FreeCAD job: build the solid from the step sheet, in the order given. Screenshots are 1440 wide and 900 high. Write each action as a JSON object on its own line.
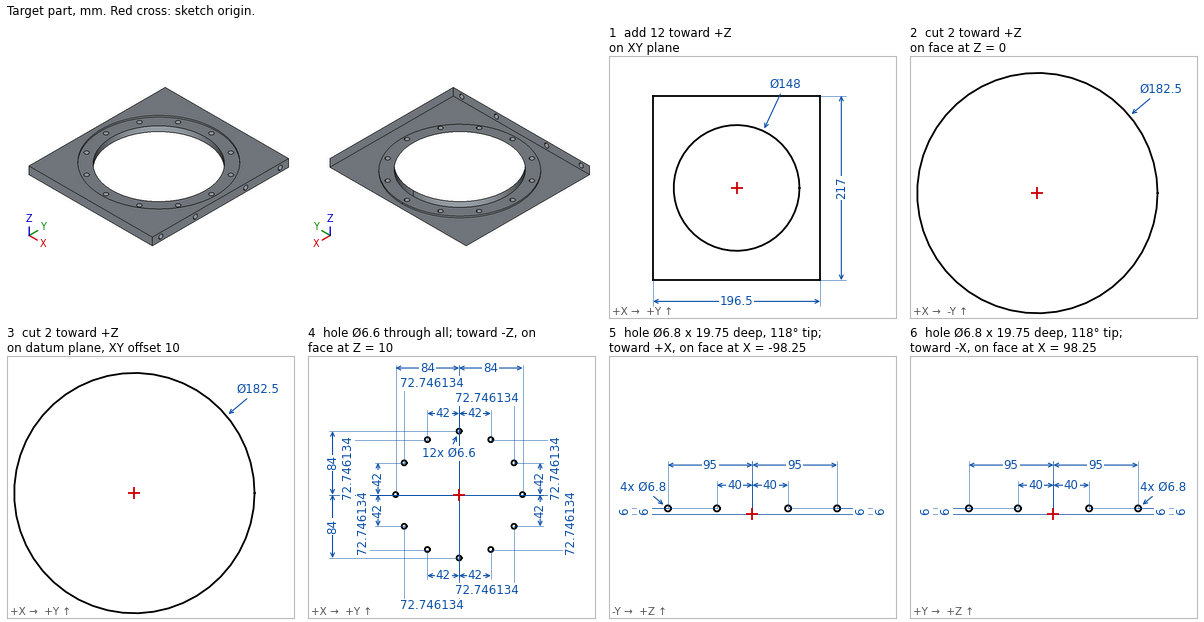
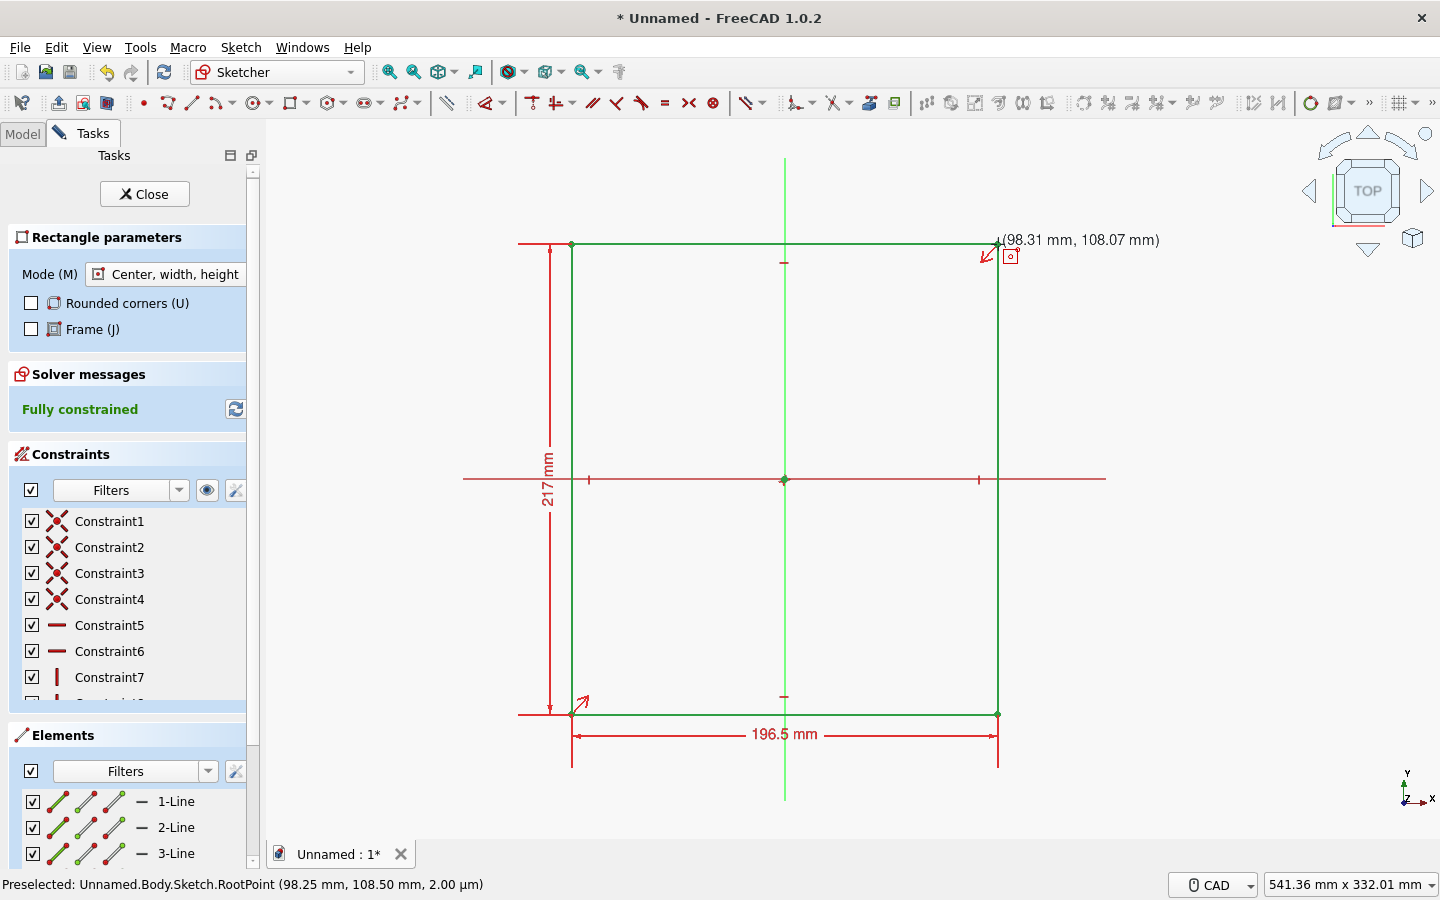
{"action": "left_click", "coordinate": [254, 104]}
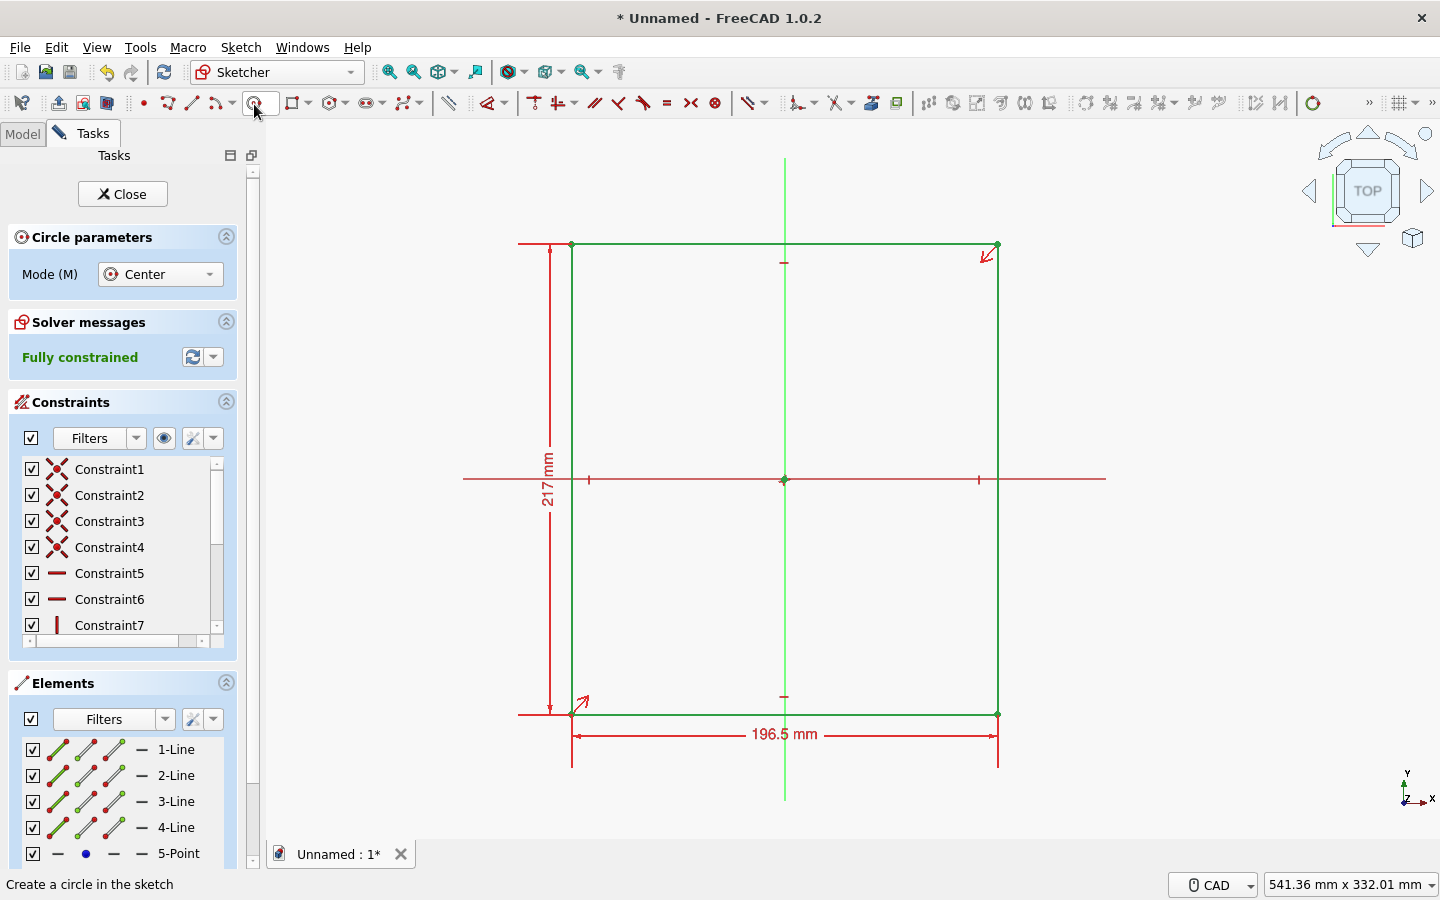
{"action": "left_click", "coordinate": [785, 479]}
{"action": "mouse_move", "coordinate": [898, 366]}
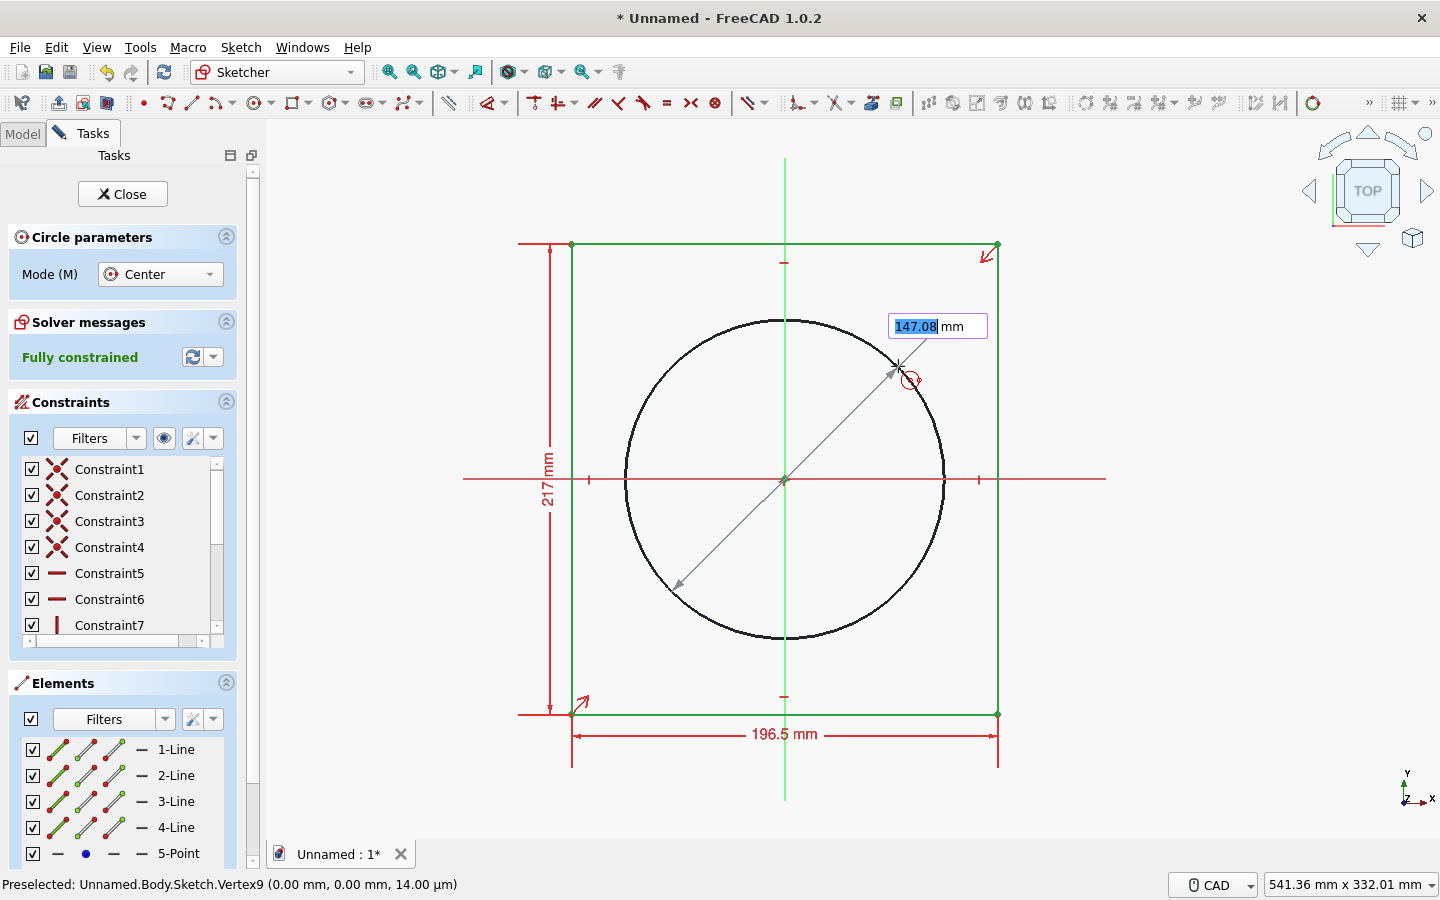
{"action": "type", "text": "148"}
{"action": "key", "text": "Return"}
{"action": "key", "text": "Escape"}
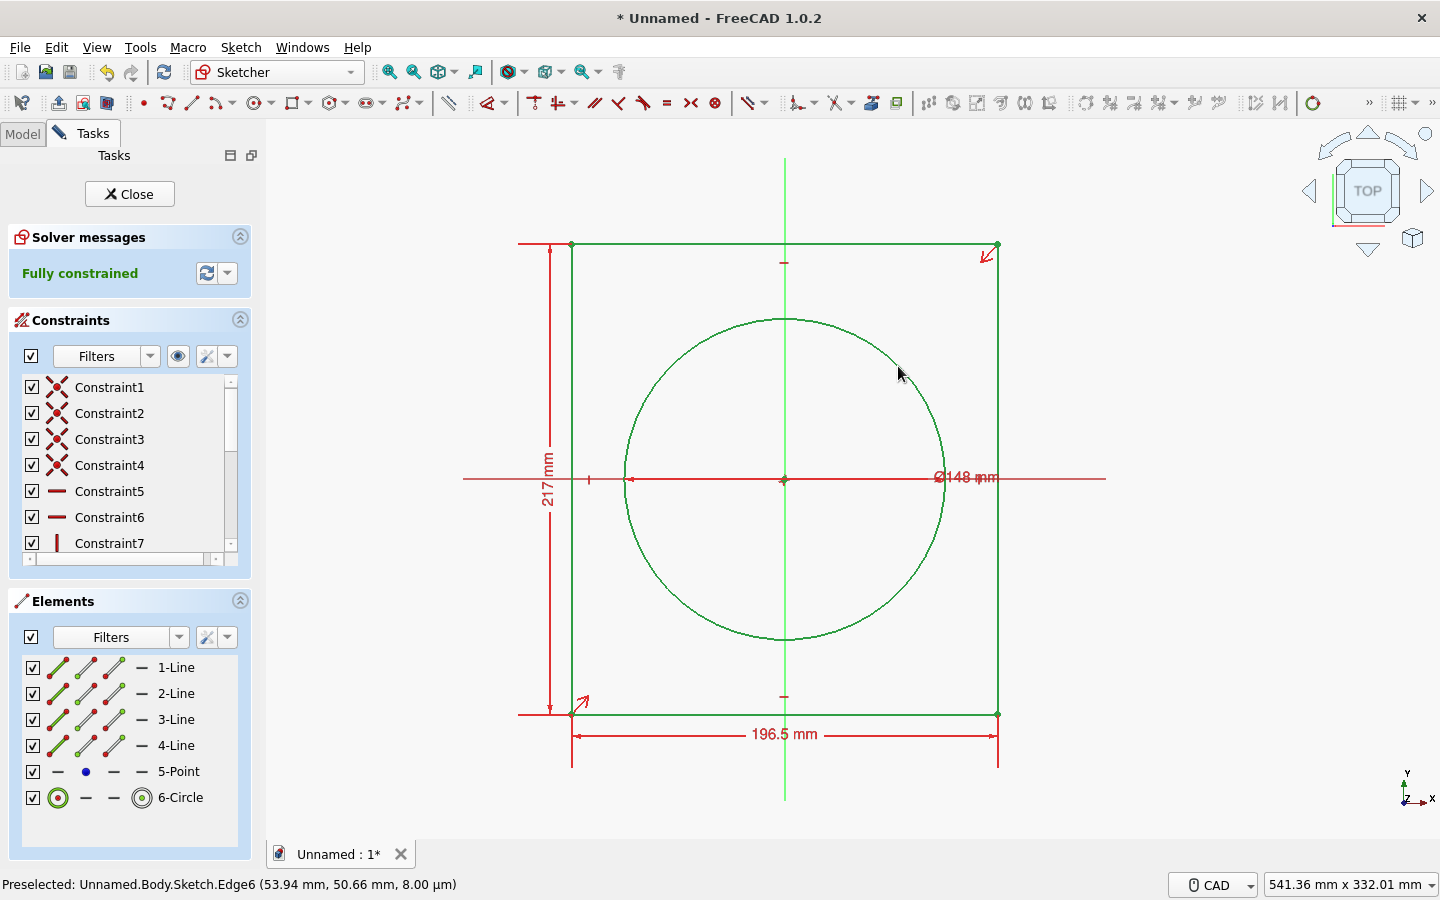
{"action": "left_click", "coordinate": [130, 194]}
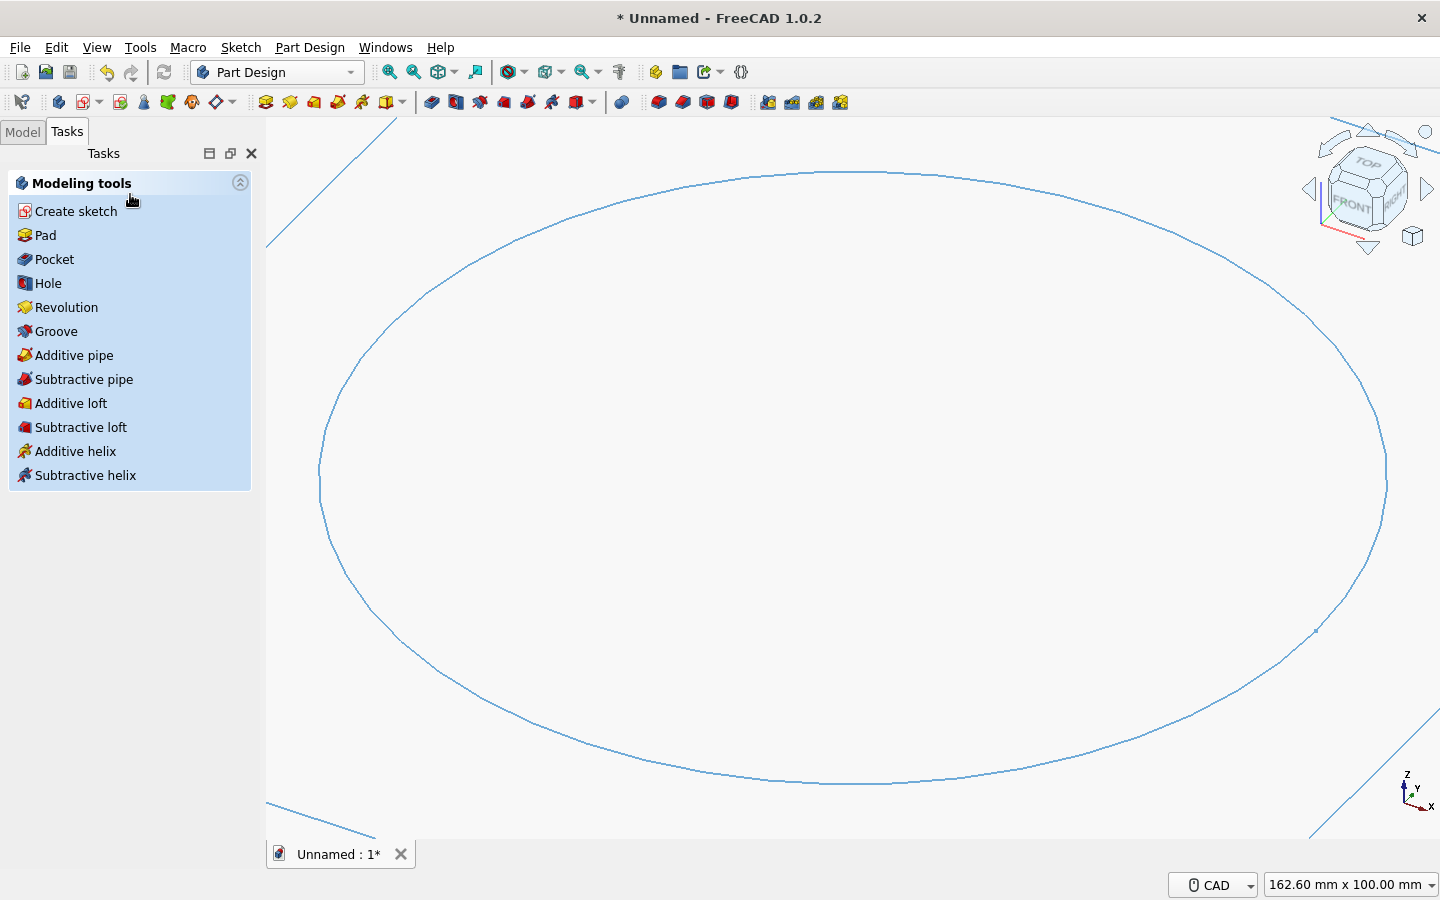
{"action": "left_click", "coordinate": [266, 102]}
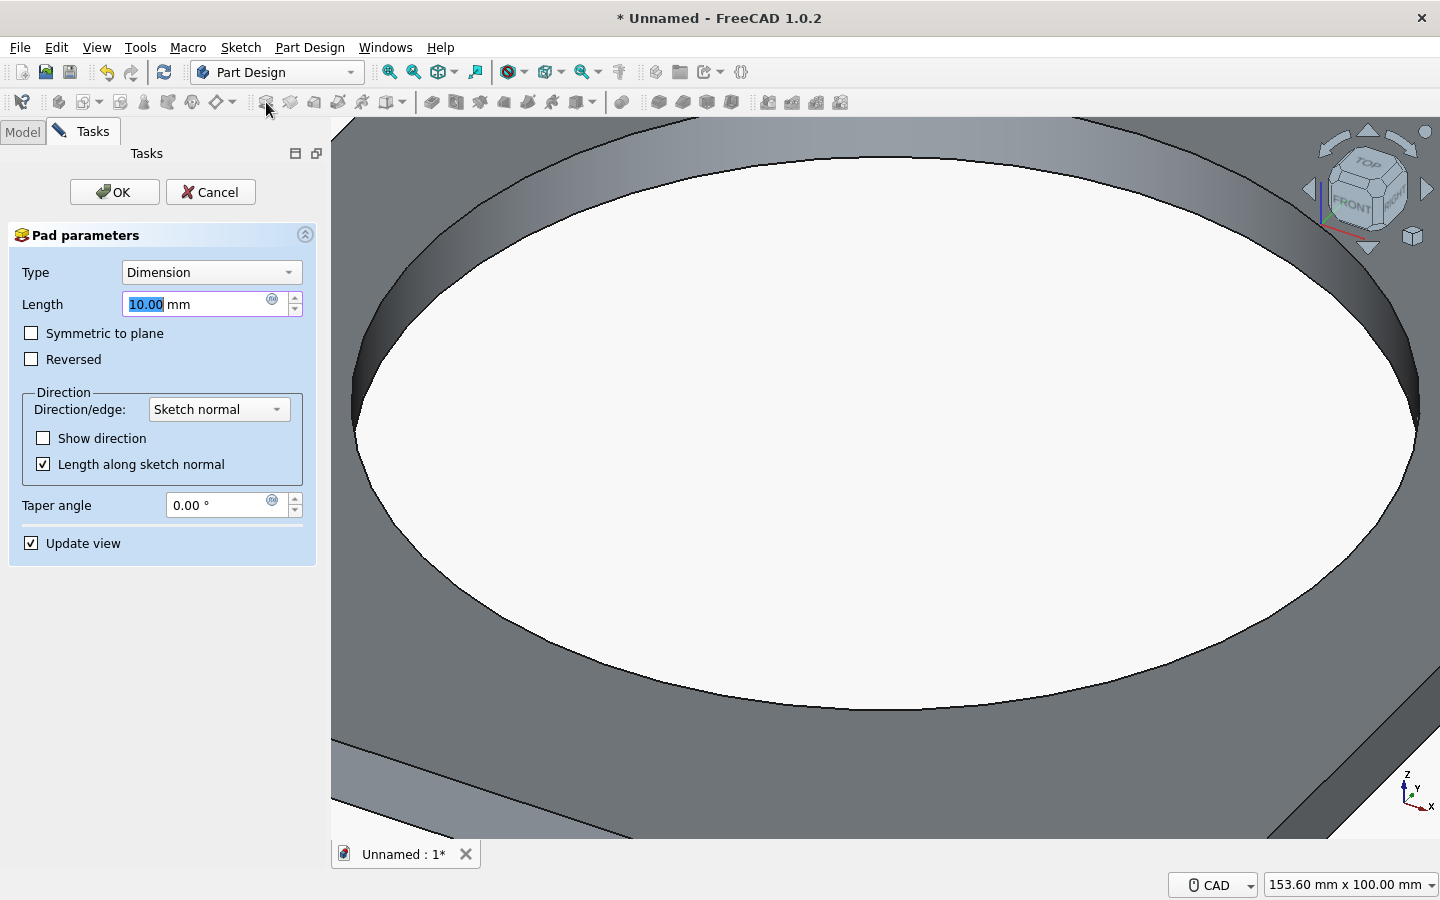
{"action": "type", "text": "12"}
{"action": "key", "text": "Tab"}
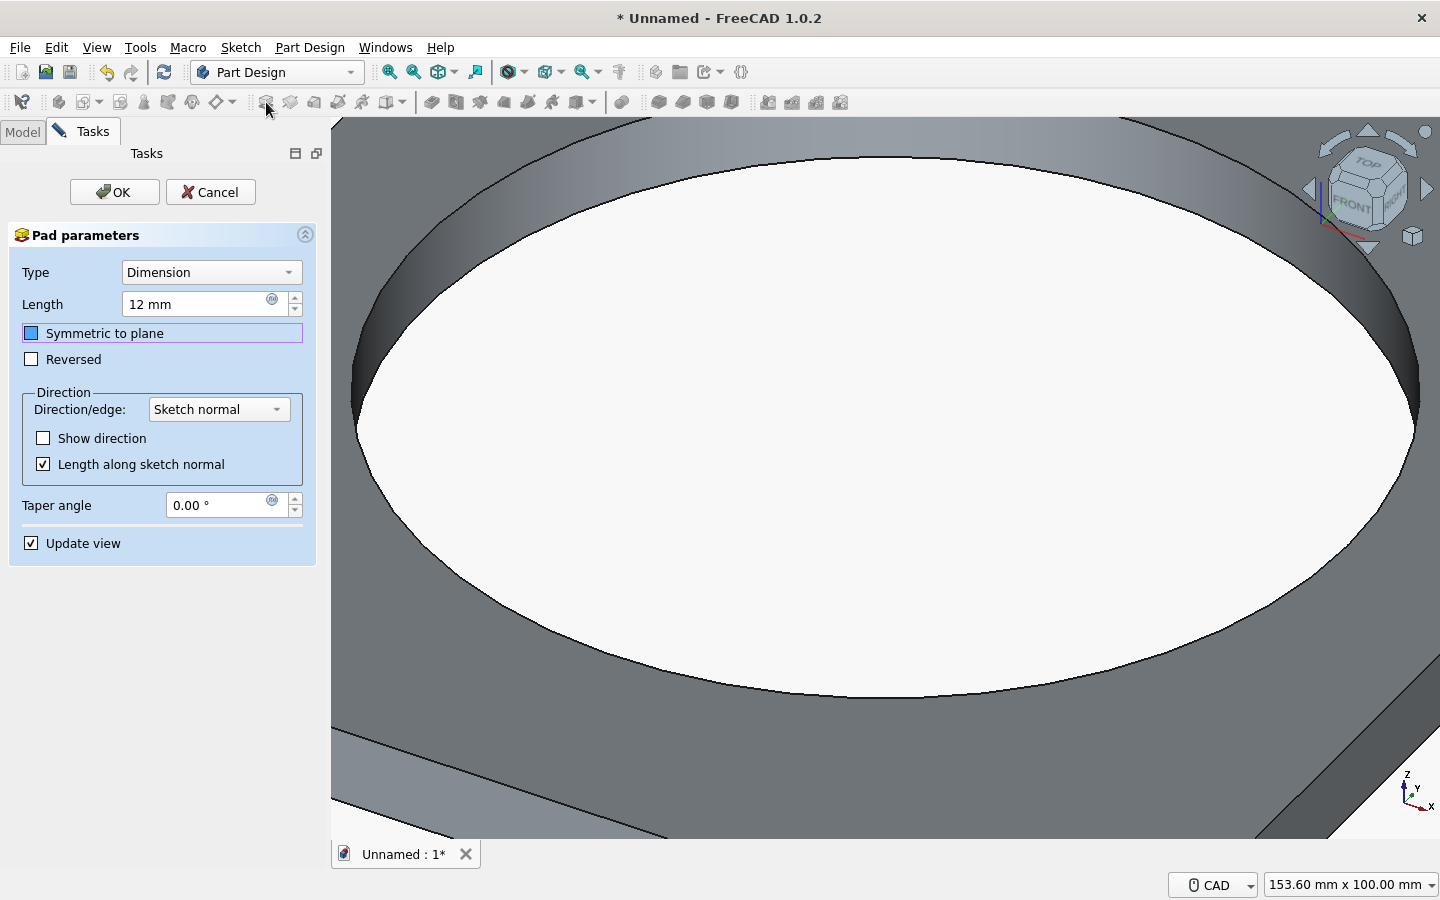
{"action": "left_click", "coordinate": [115, 192]}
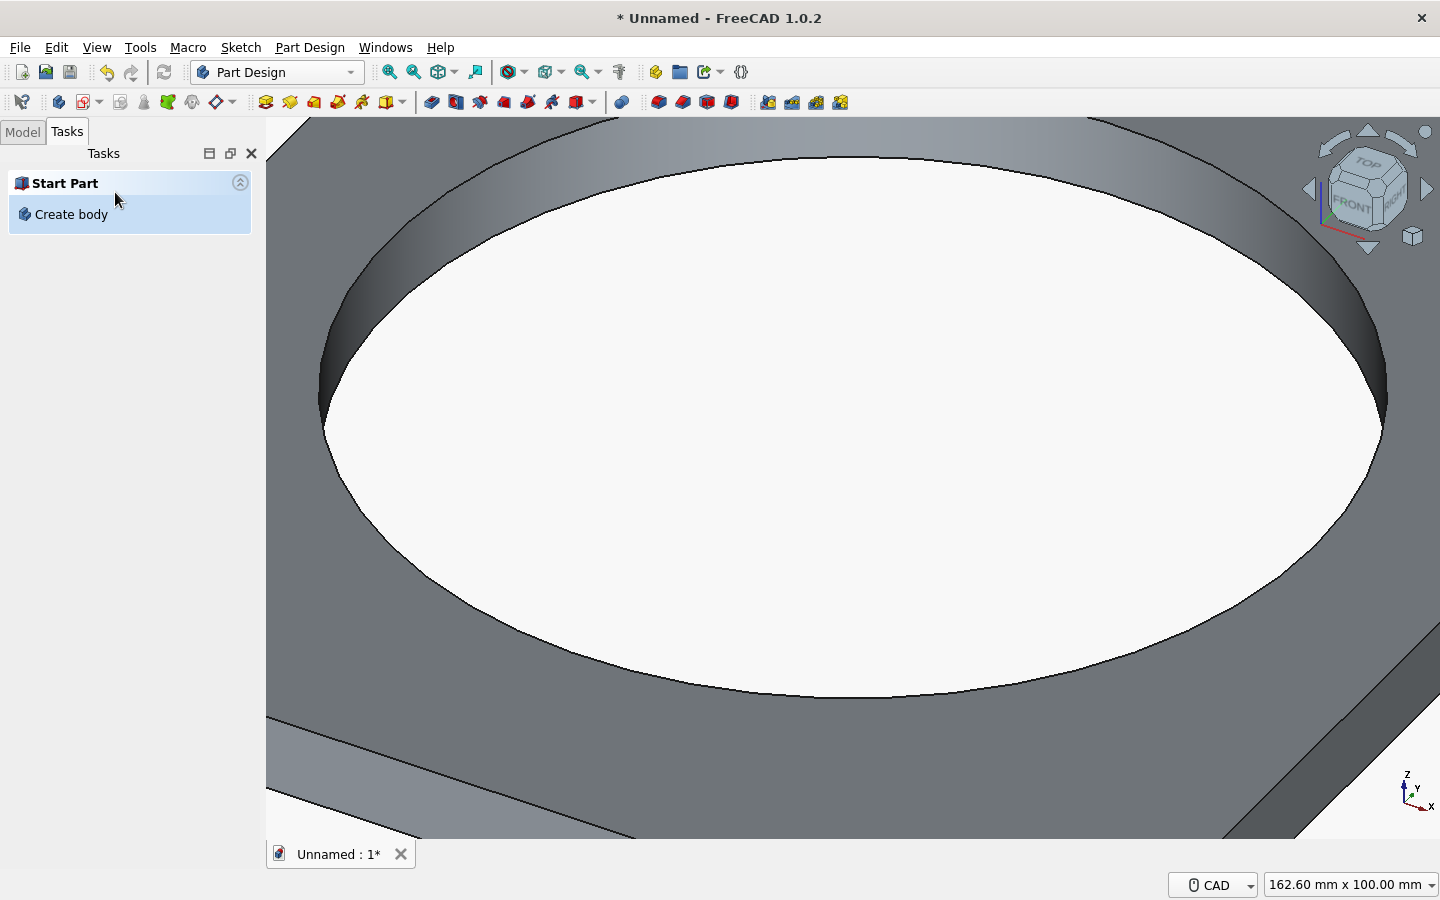
{"action": "left_click", "coordinate": [390, 72]}